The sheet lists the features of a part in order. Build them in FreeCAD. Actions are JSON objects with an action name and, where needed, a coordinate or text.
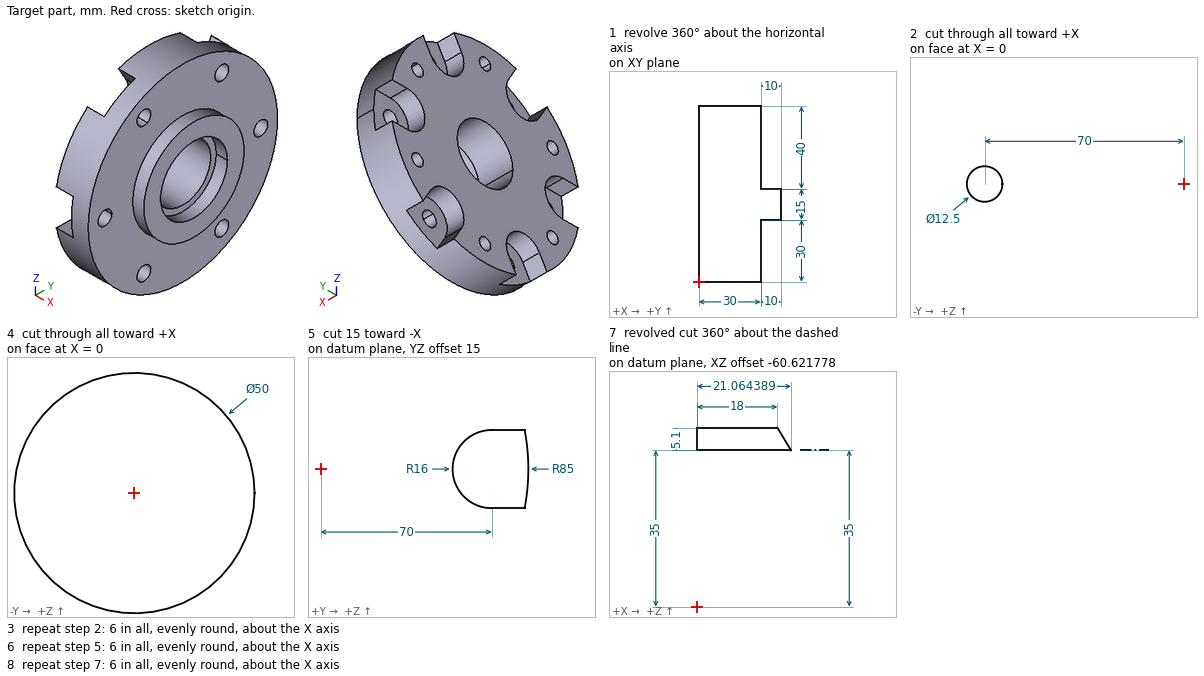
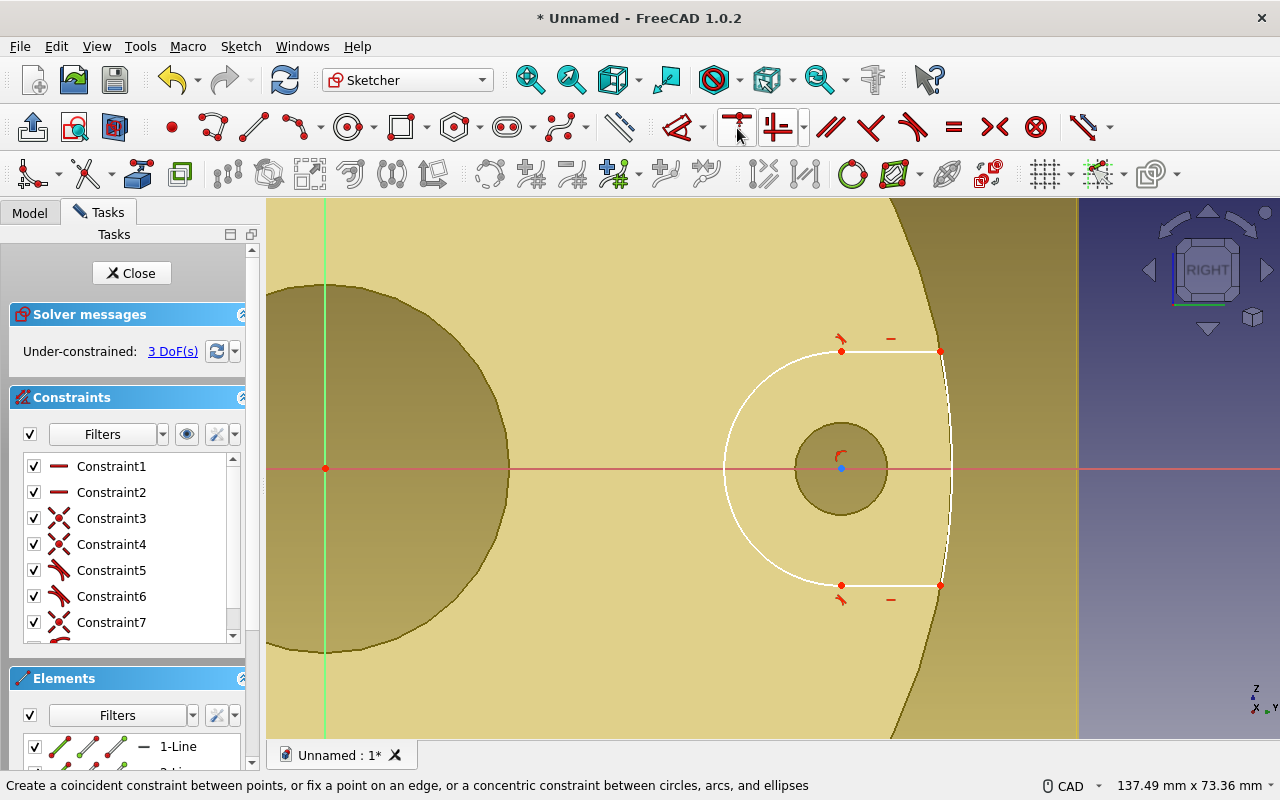
{"action": "left_click", "coordinate": [676, 128]}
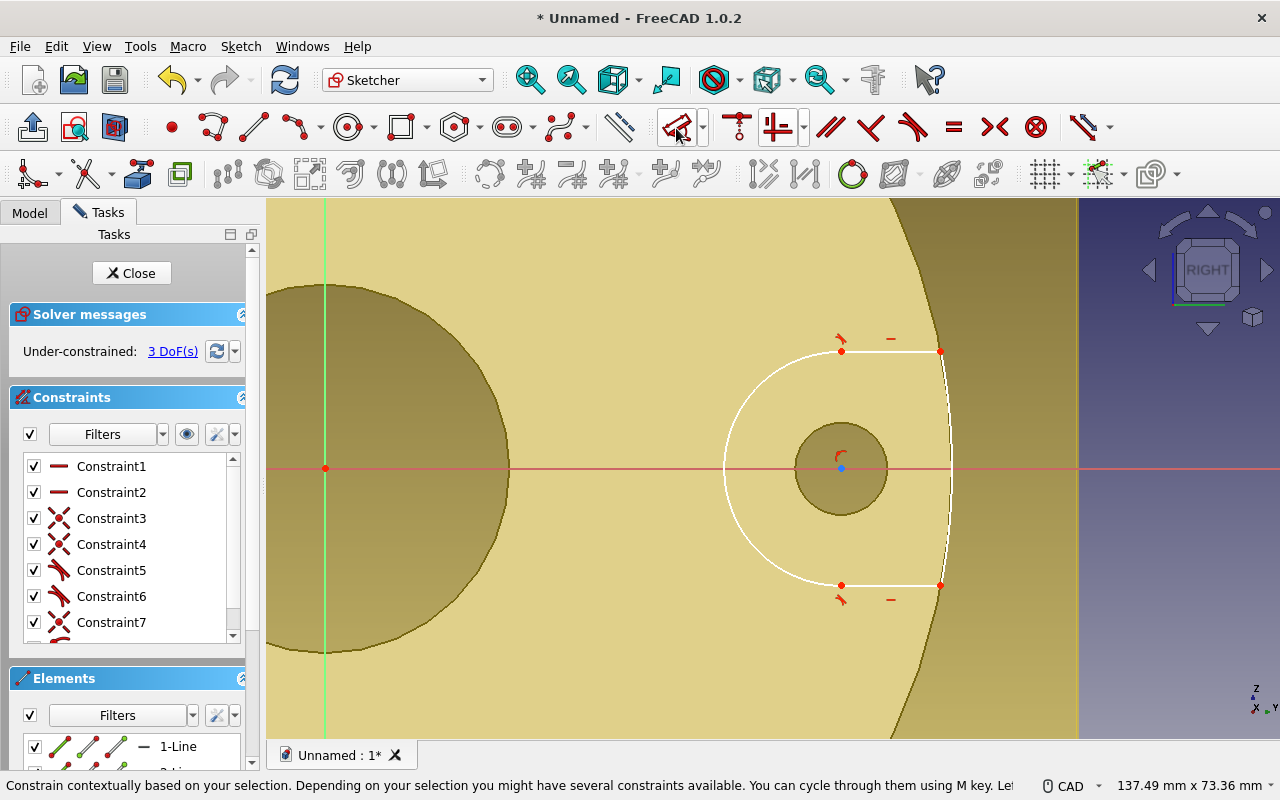
{"action": "left_click", "coordinate": [747, 400]}
{"action": "left_click", "coordinate": [721, 381]}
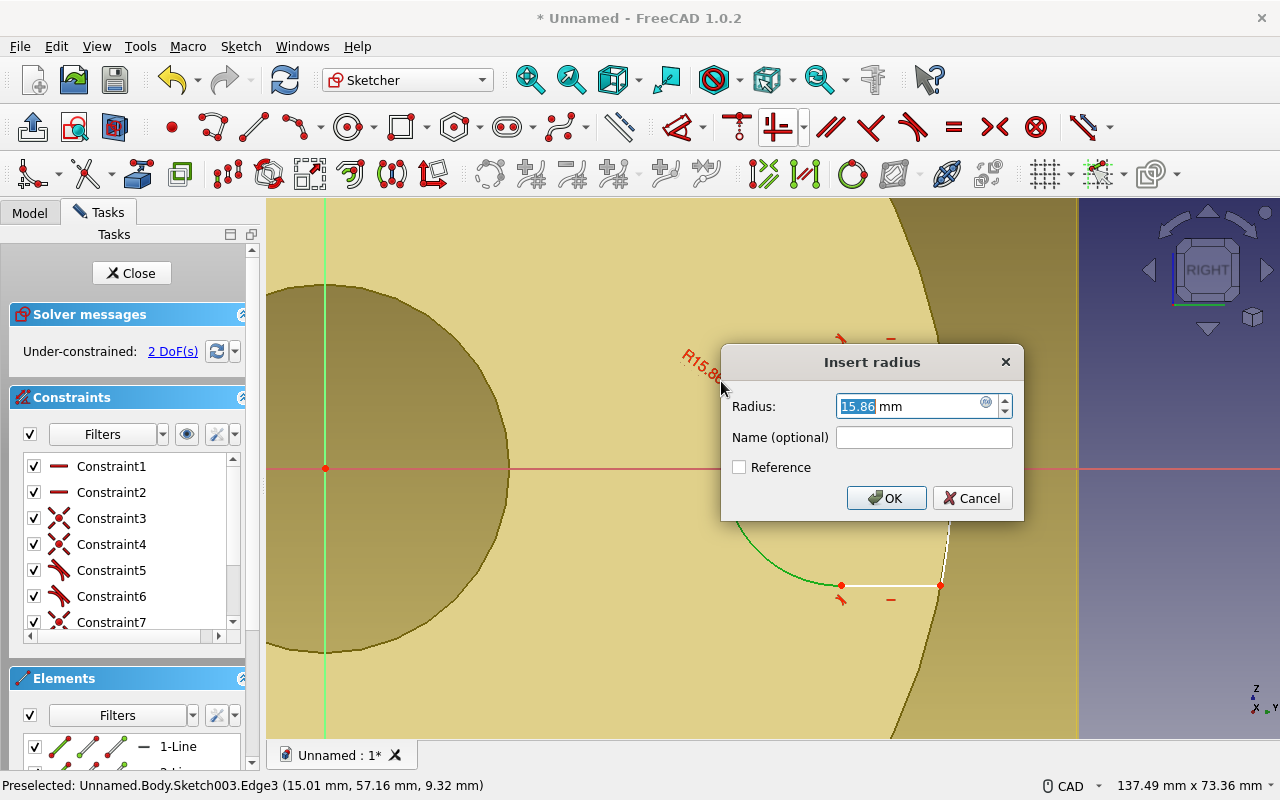
{"action": "type", "text": "16"}
{"action": "key", "text": "Return"}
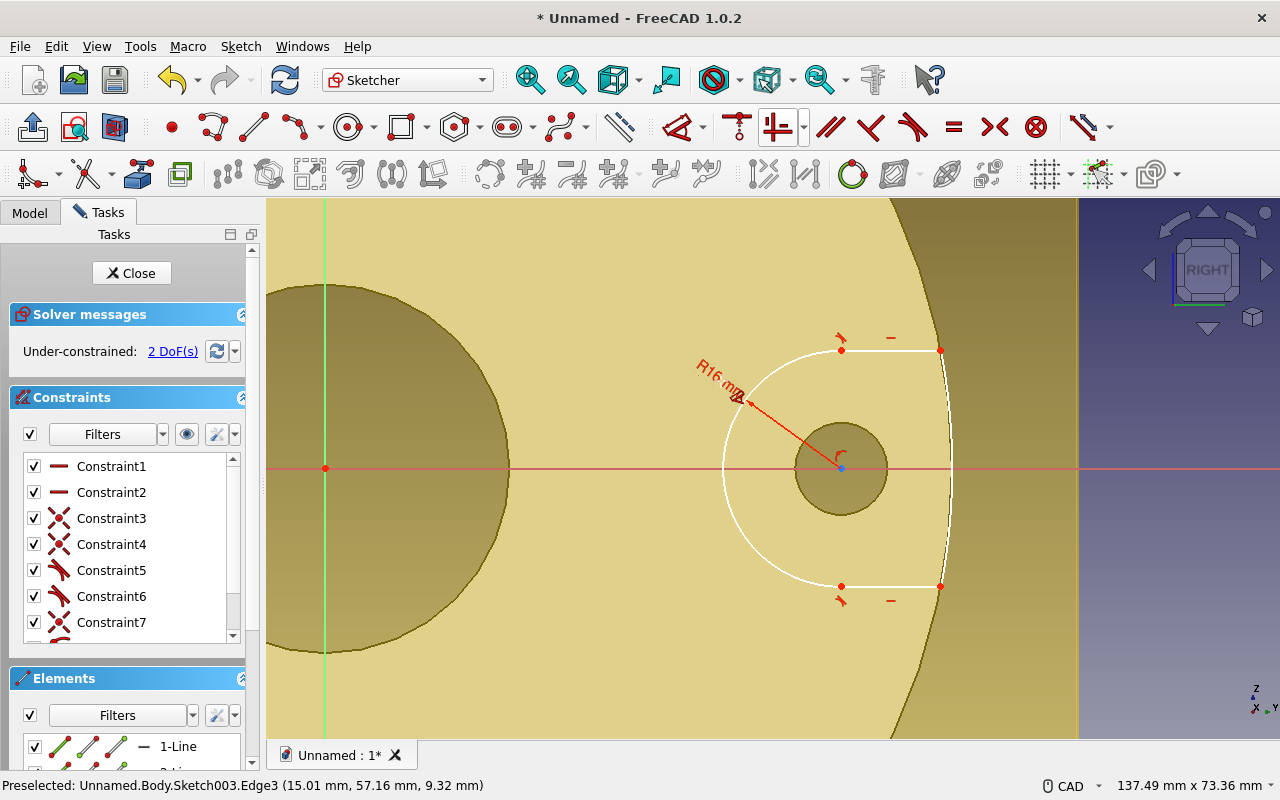
{"action": "left_click", "coordinate": [950, 516]}
{"action": "left_click", "coordinate": [982, 518]}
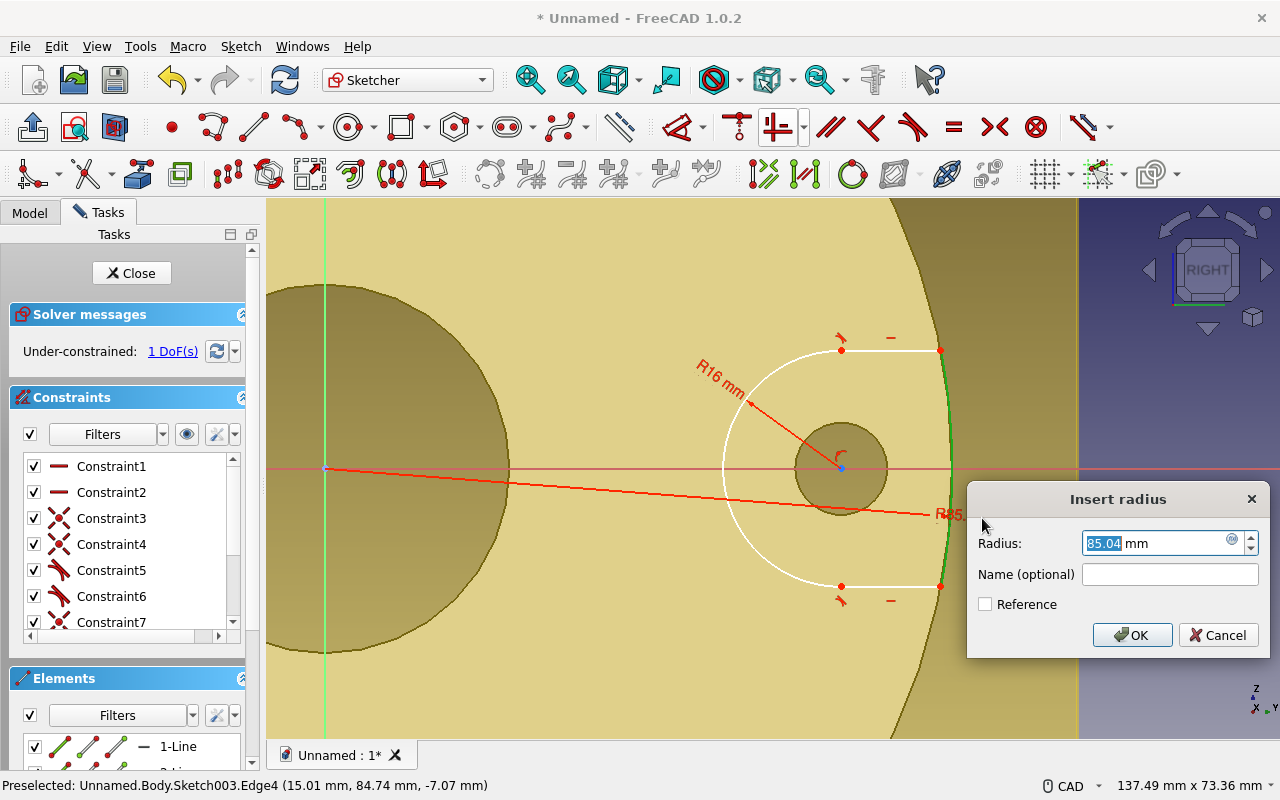
{"action": "type", "text": "85"}
{"action": "key", "text": "Return"}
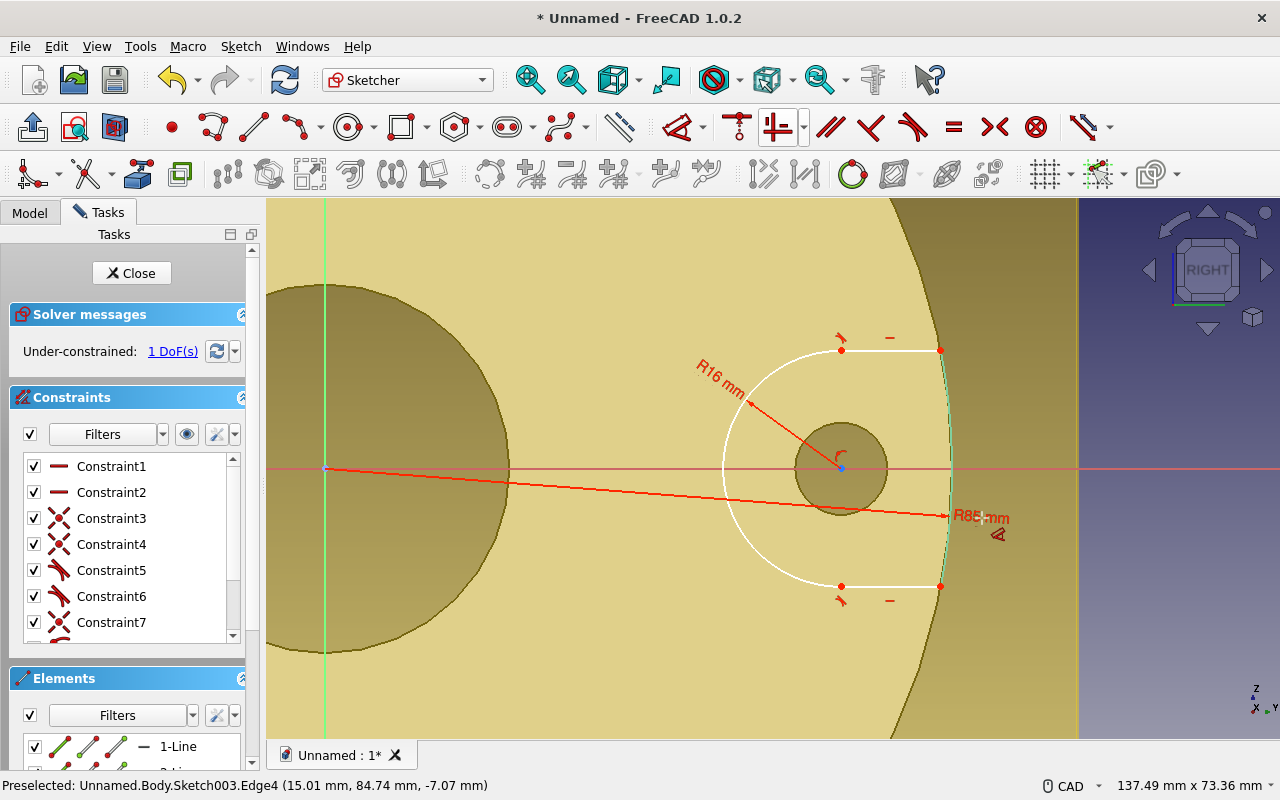
{"action": "left_click", "coordinate": [841, 587]}
{"action": "left_click", "coordinate": [583, 621]}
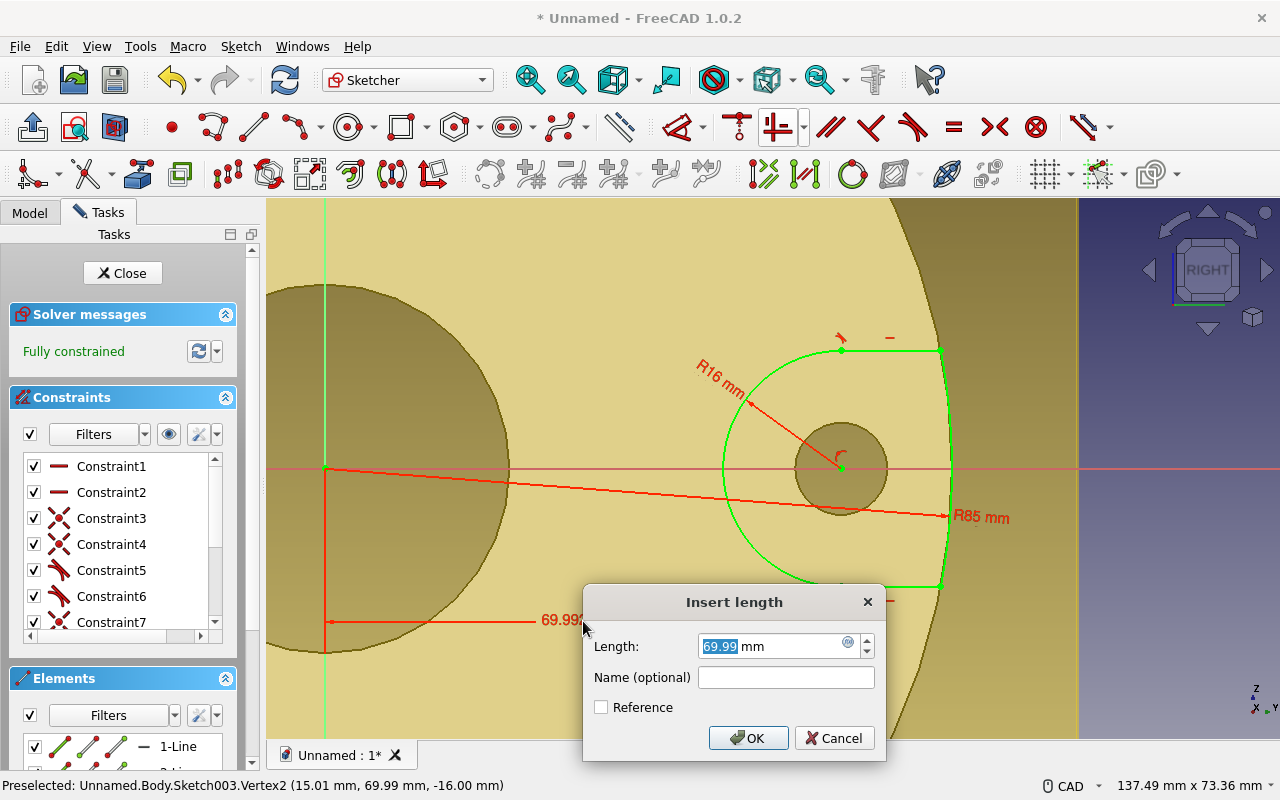
{"action": "type", "text": "70"}
{"action": "key", "text": "Return"}
{"action": "key", "text": "Escape"}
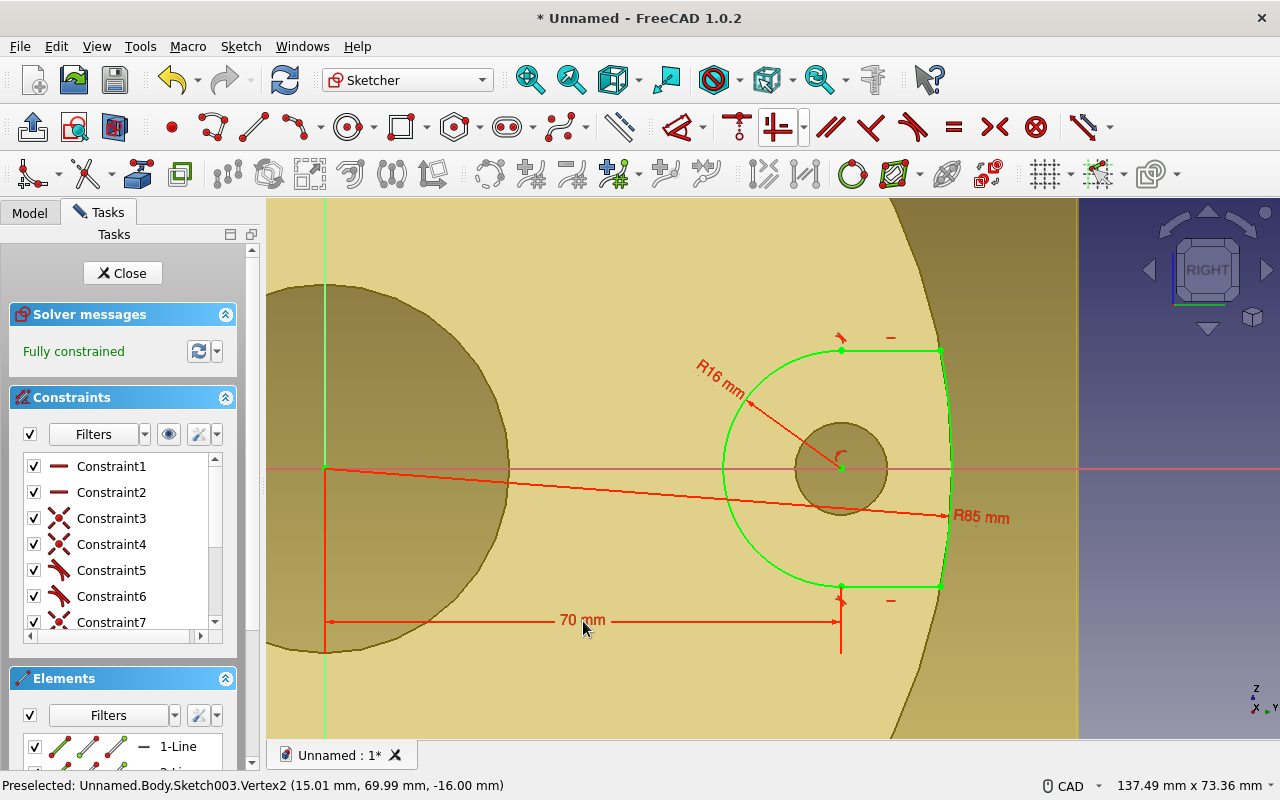
{"action": "left_click", "coordinate": [123, 273]}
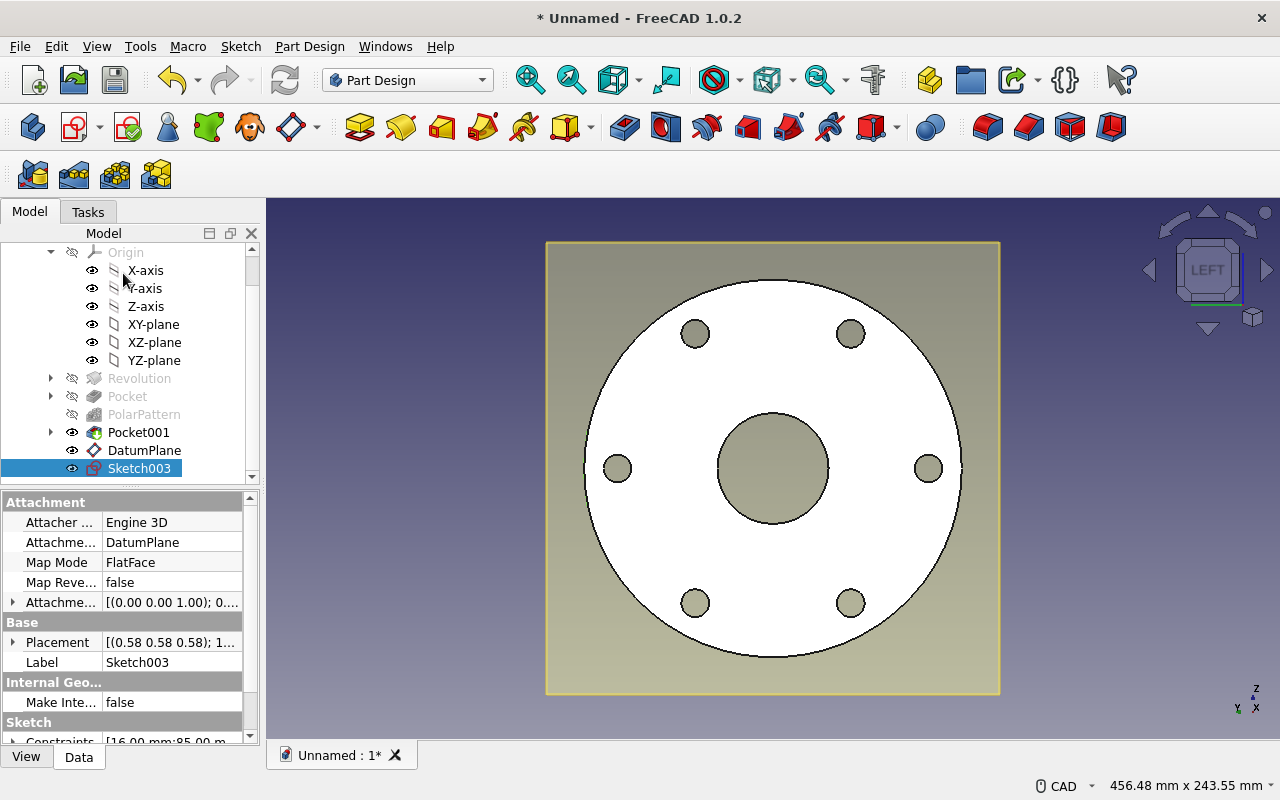
{"action": "left_click", "coordinate": [625, 128]}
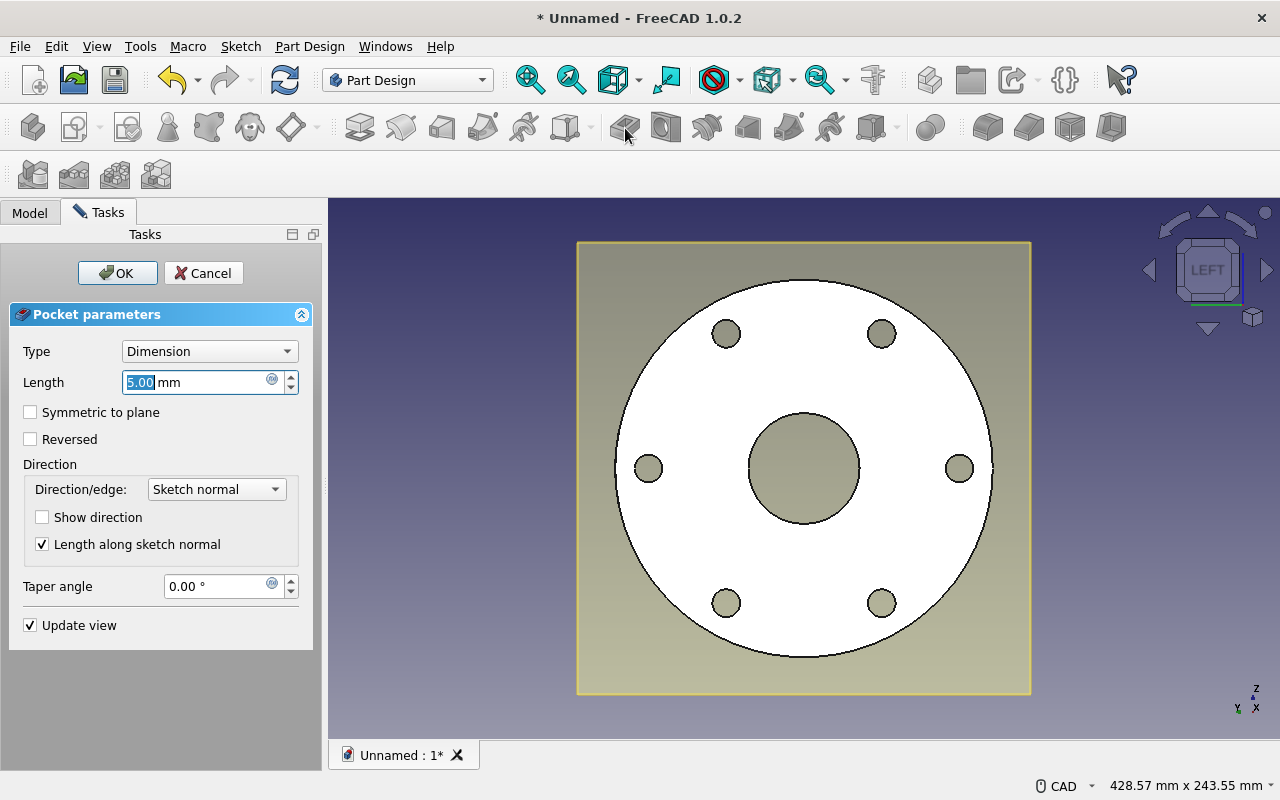
{"action": "type", "text": "15"}
{"action": "key", "text": "Tab"}